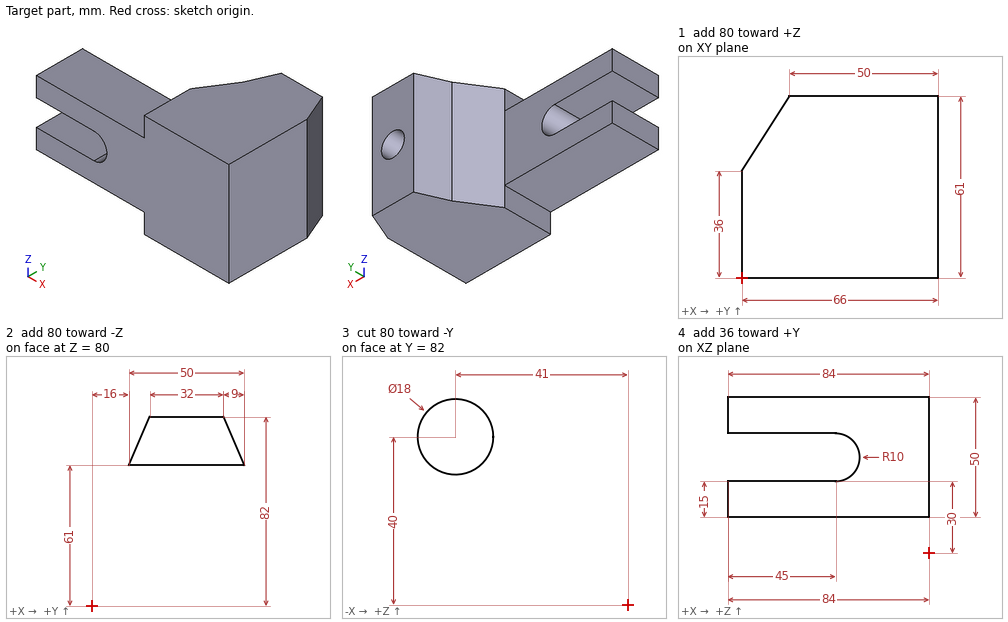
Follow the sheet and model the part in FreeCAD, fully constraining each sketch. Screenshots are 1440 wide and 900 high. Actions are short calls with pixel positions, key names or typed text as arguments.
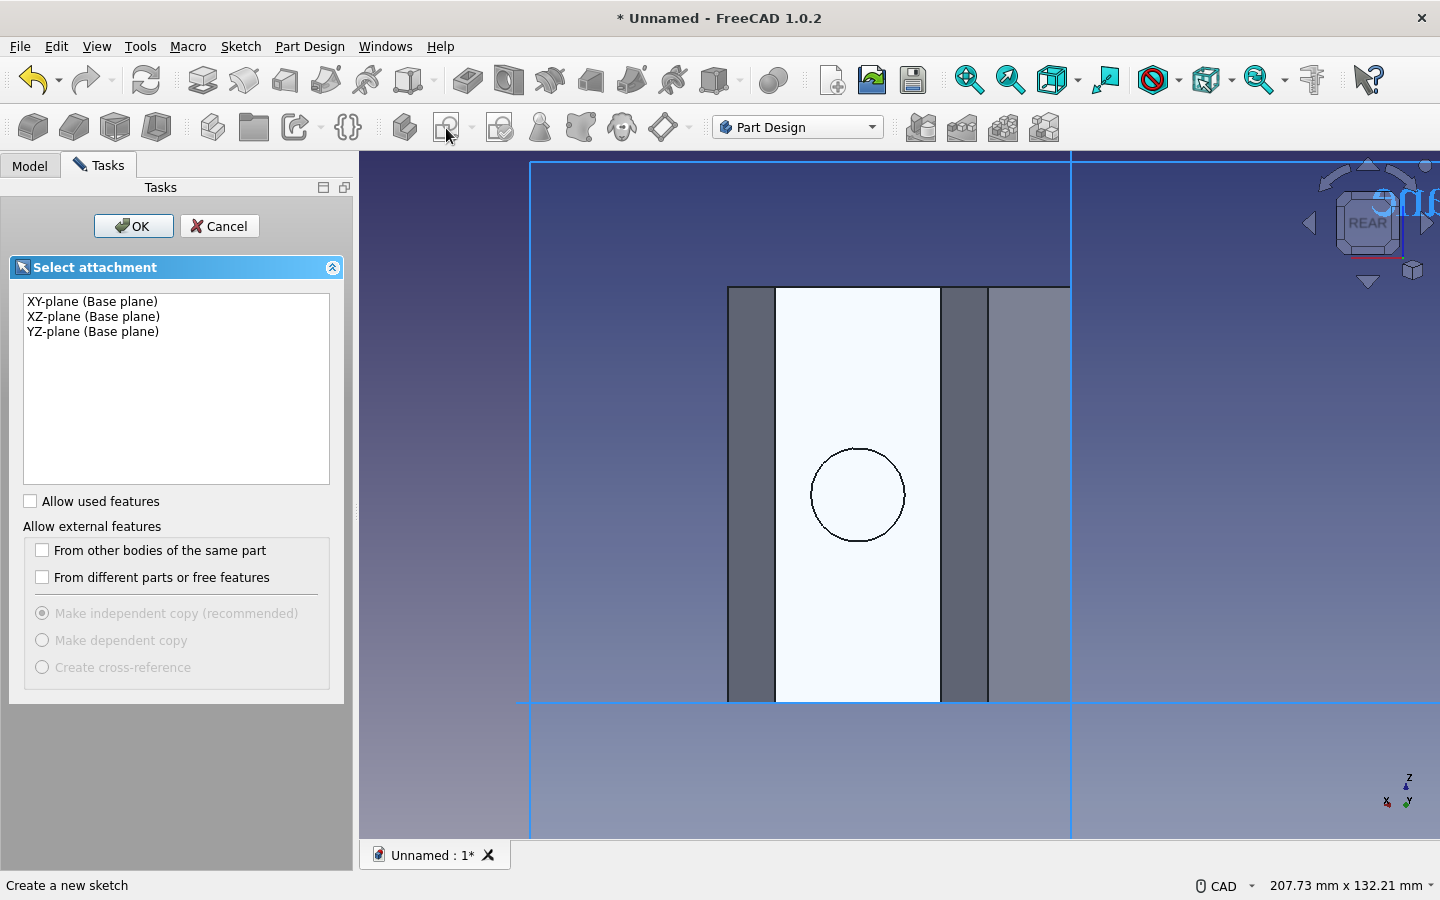
click(84, 316)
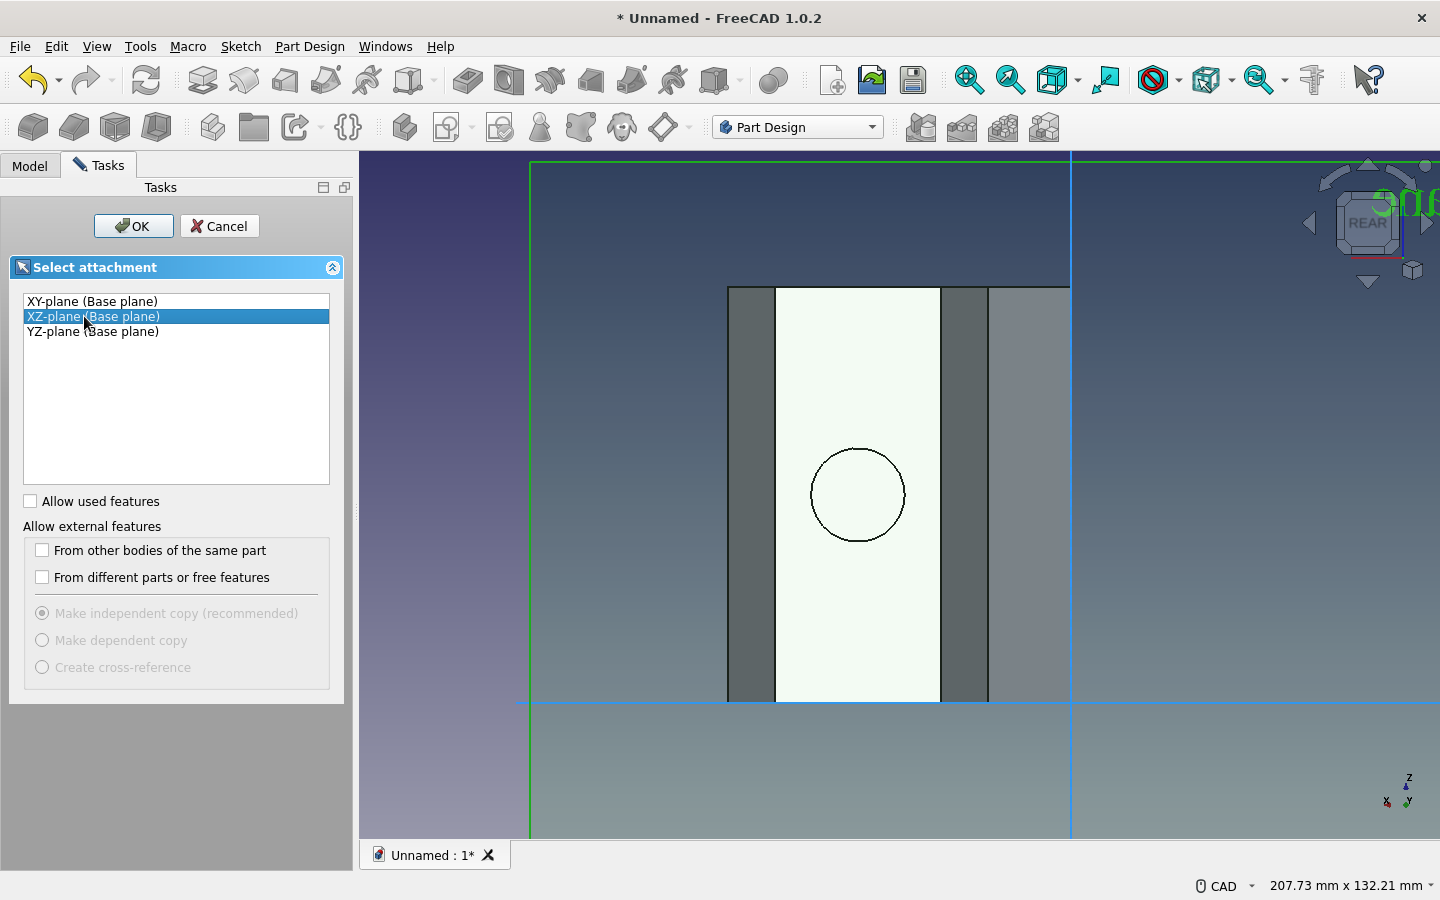
click(134, 226)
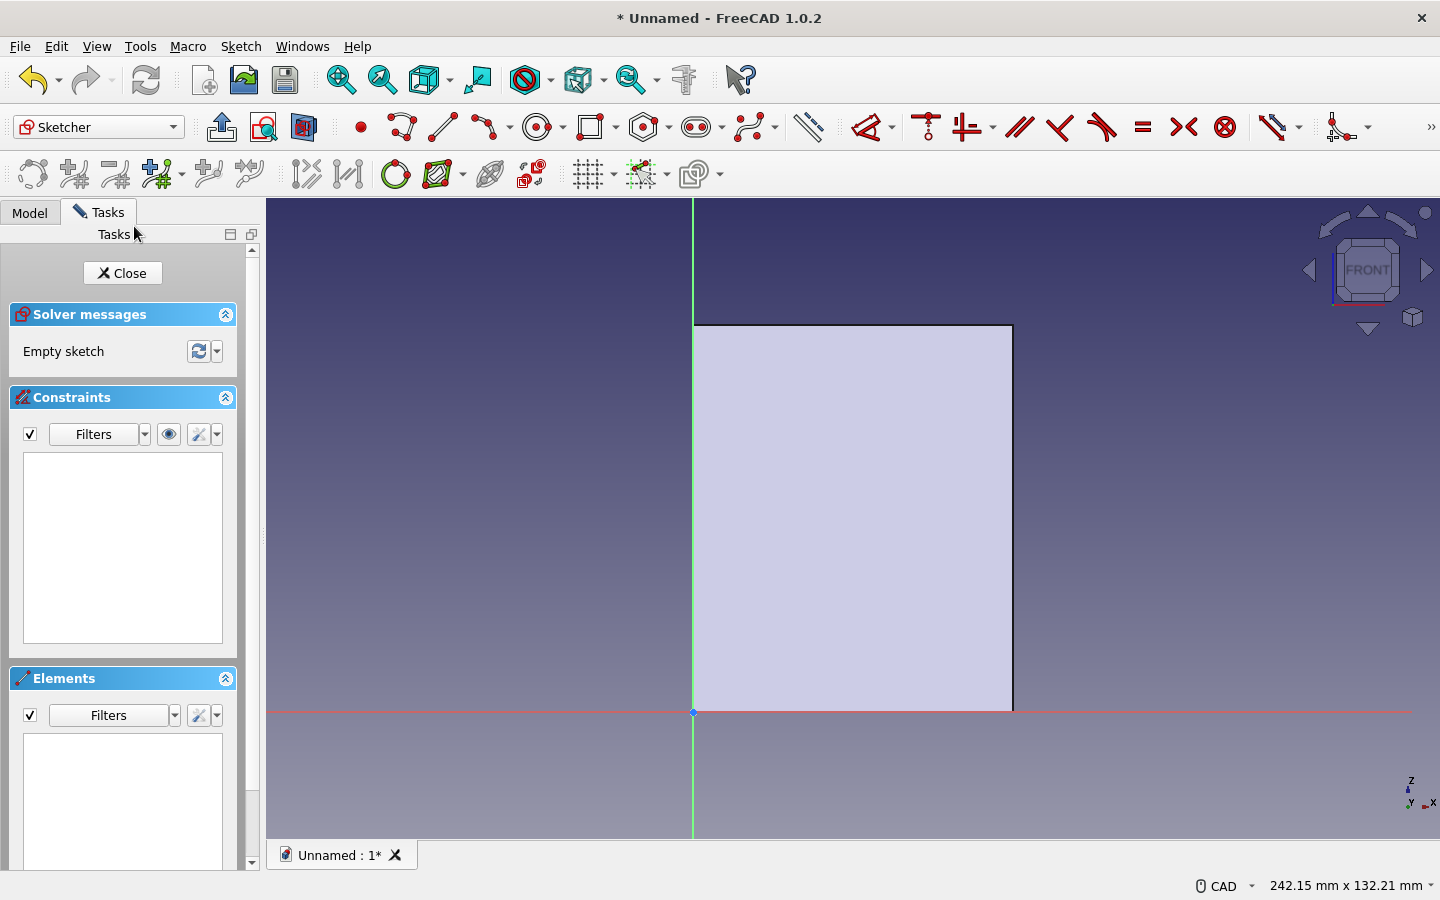
scroll(1275, 354, down, 1)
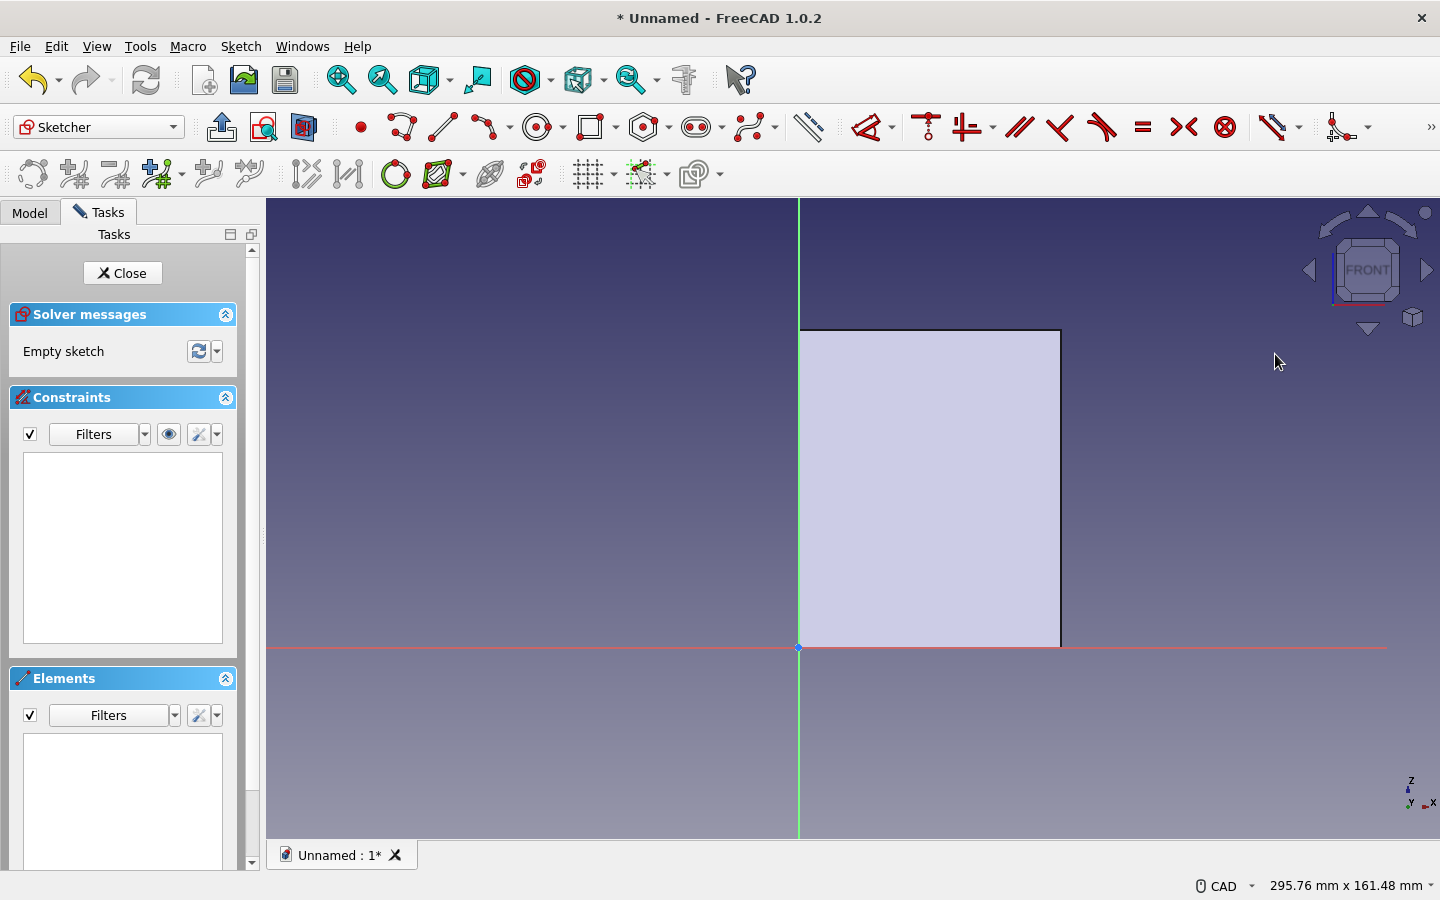
scroll(322, 518, up, 2)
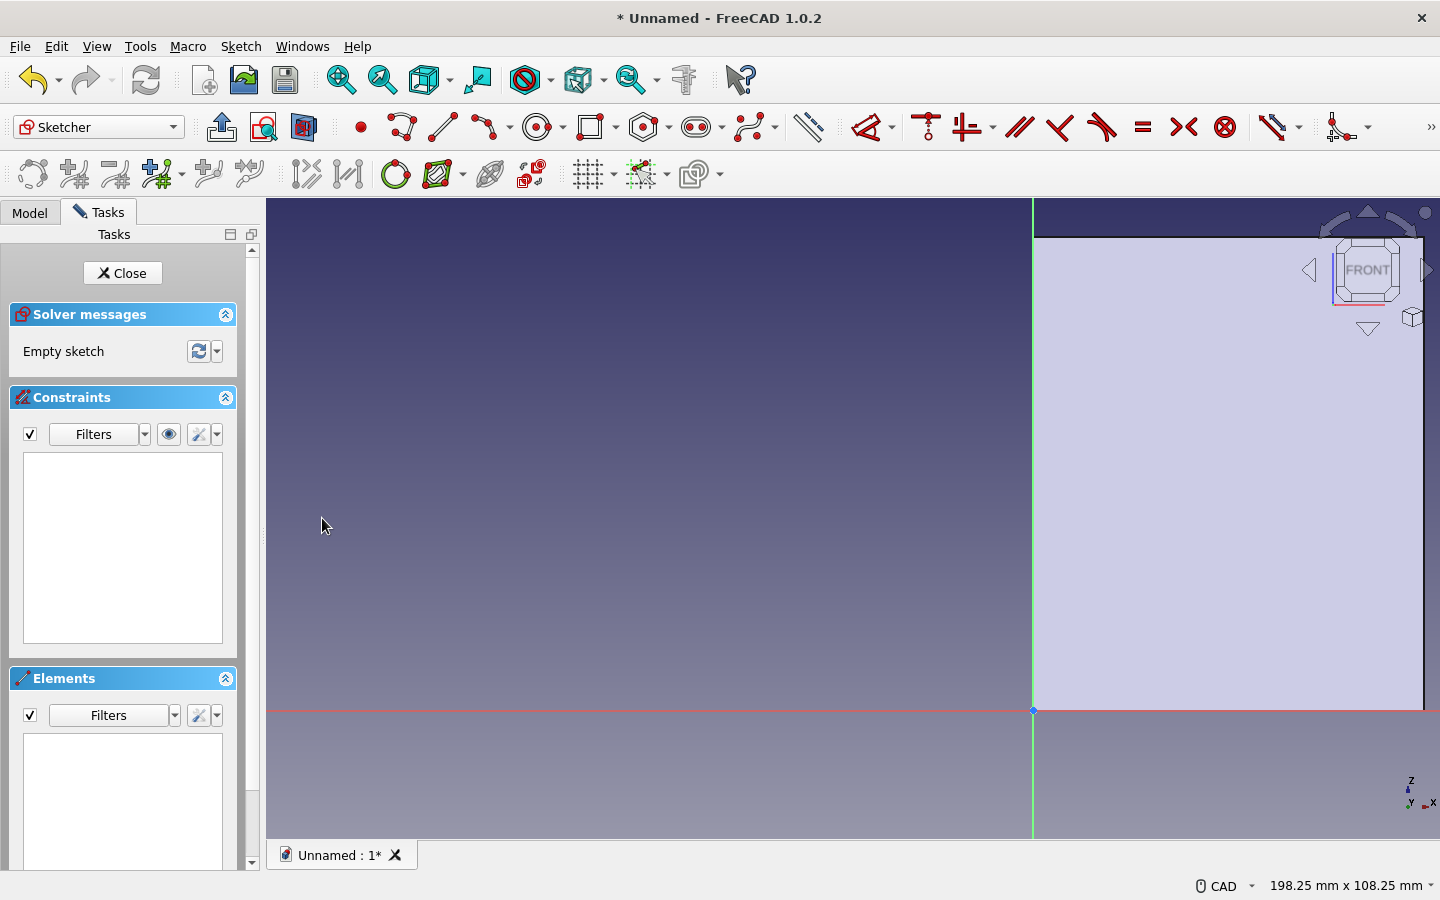
key(g)
key(m)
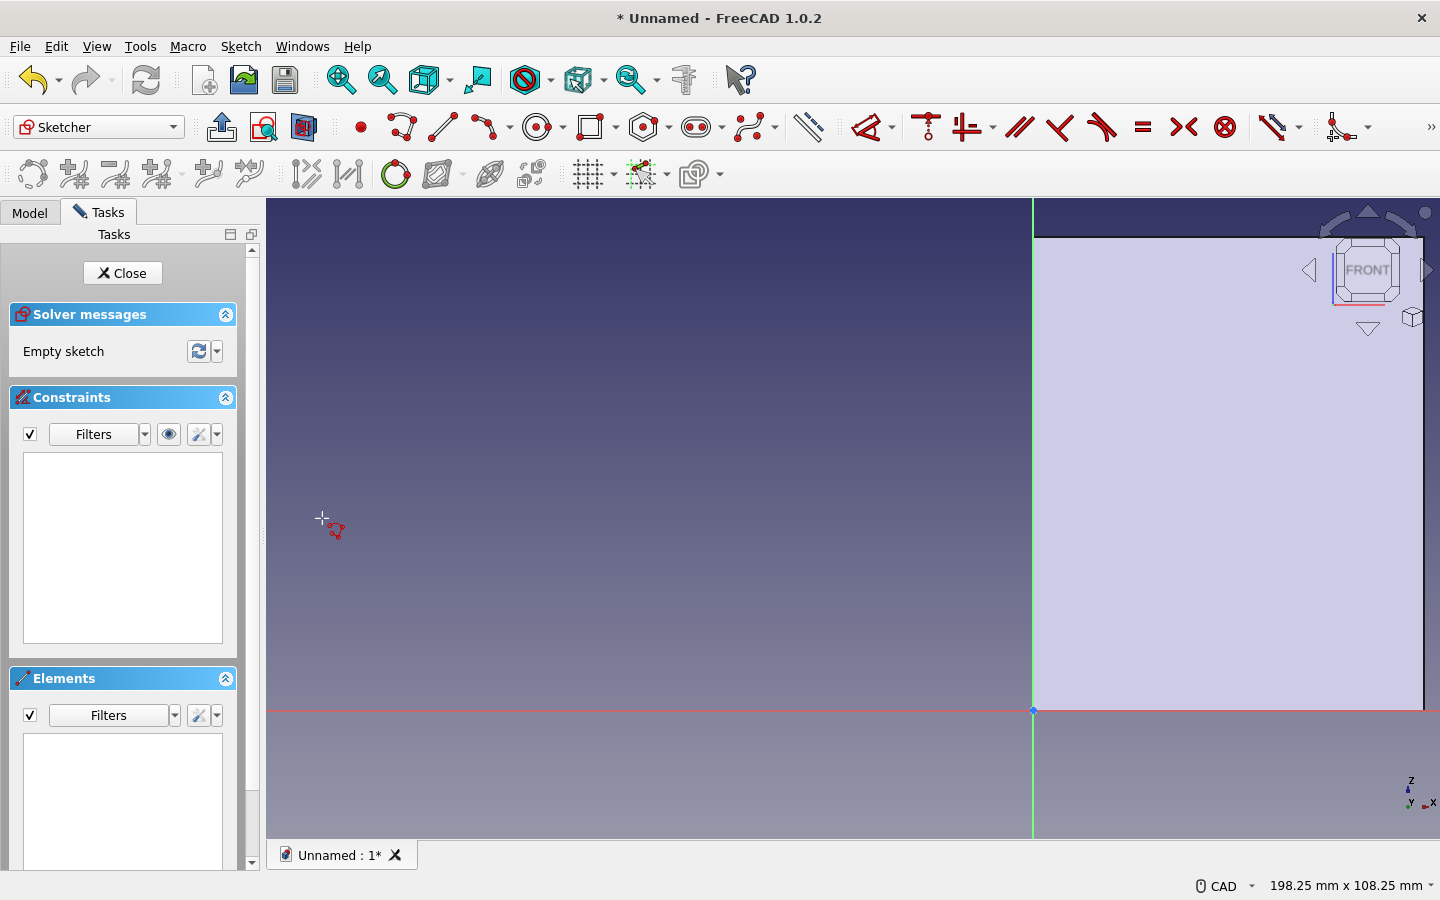
click(802, 533)
click(536, 533)
click(536, 622)
click(1033, 622)
click(1024, 326)
click(536, 326)
click(536, 415)
click(802, 415)
right_click(802, 415)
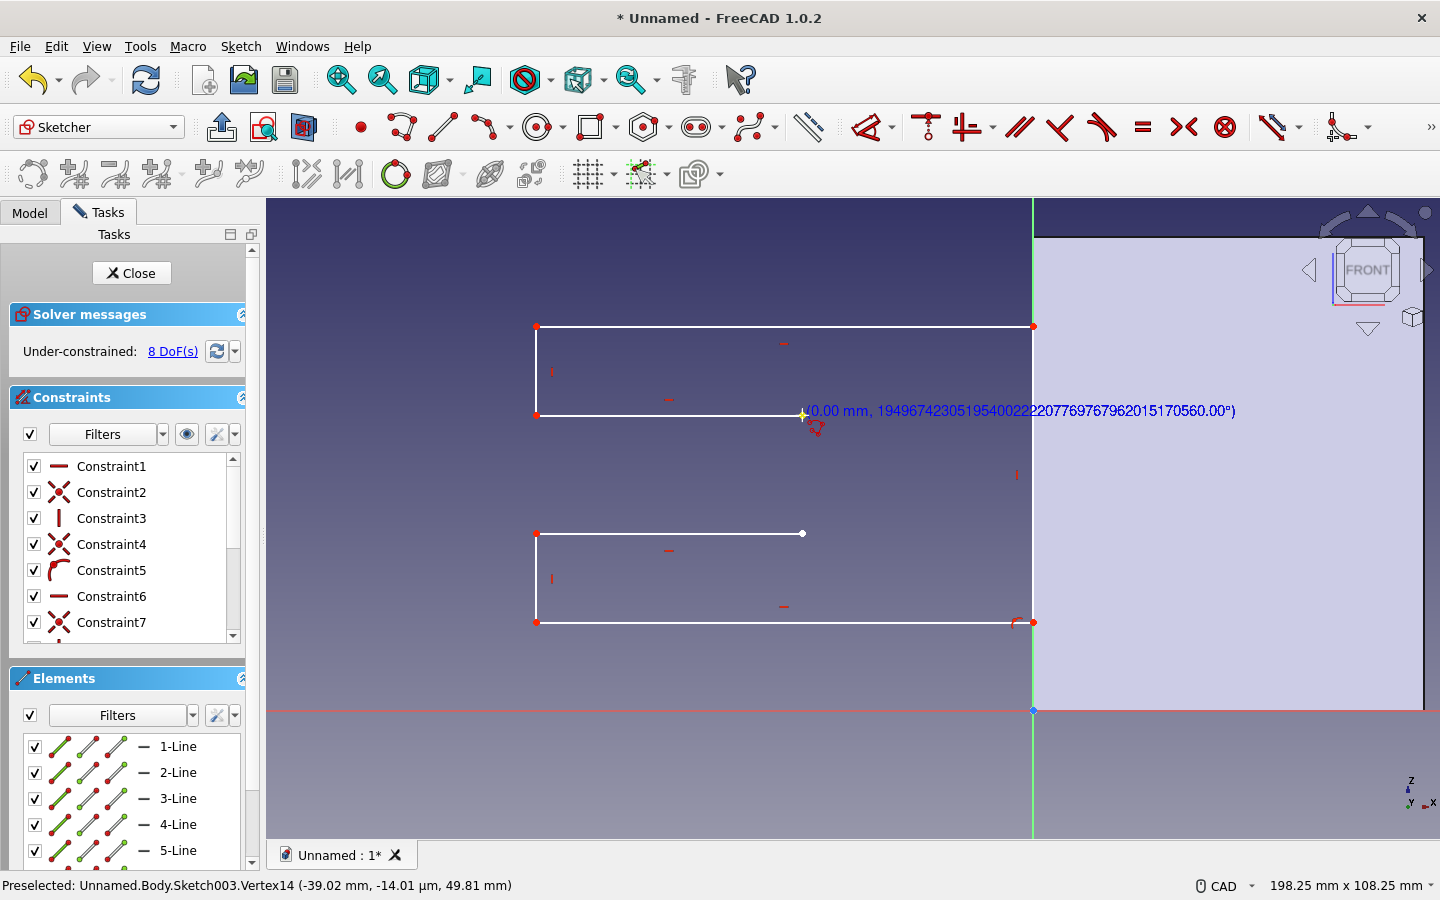
click(484, 128)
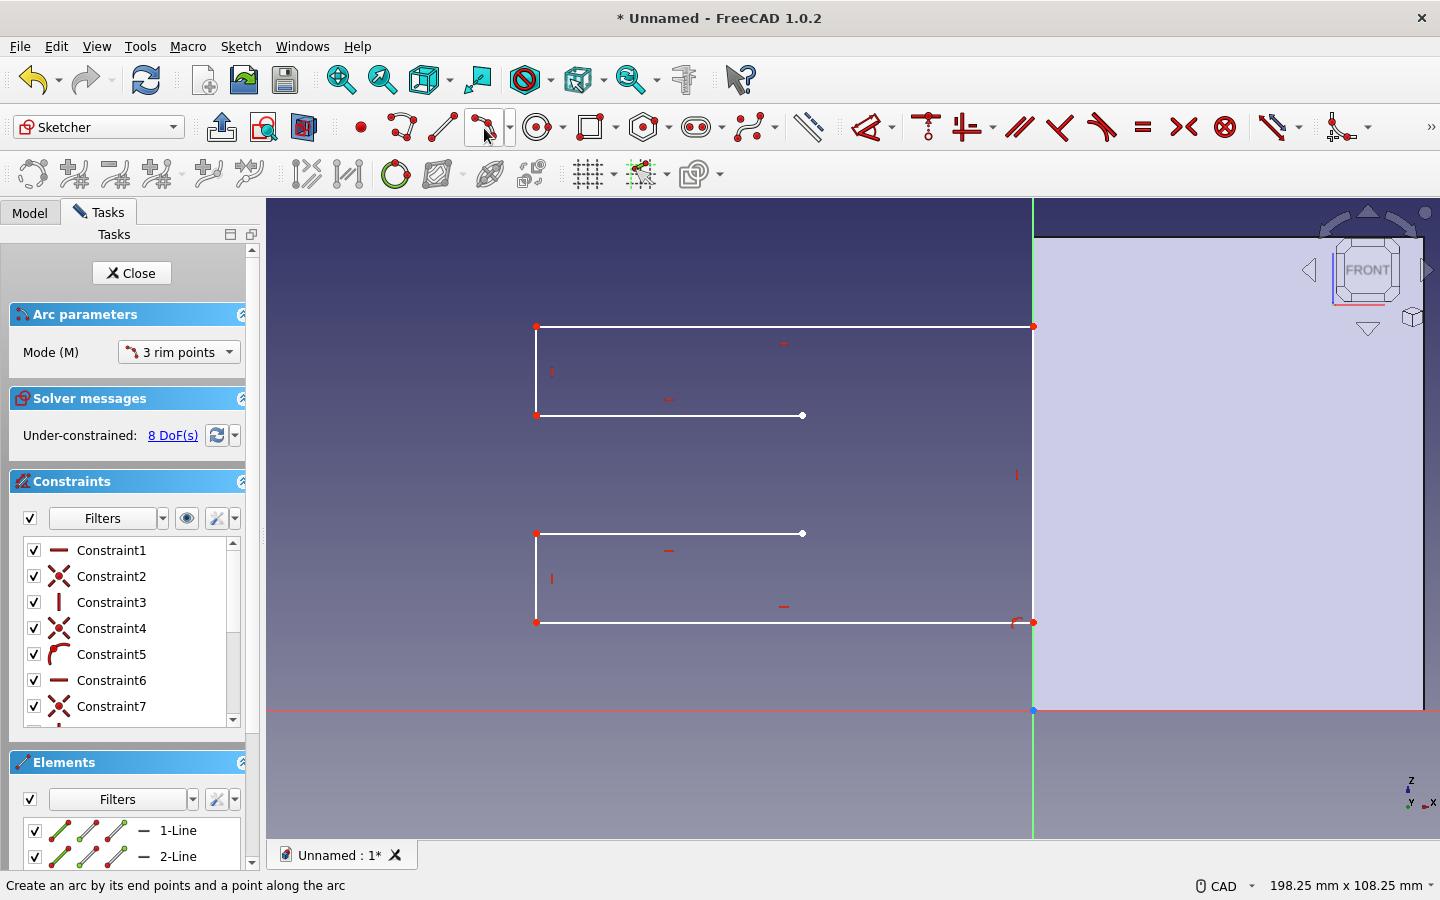
click(802, 416)
click(802, 534)
click(861, 474)
key(Escape)